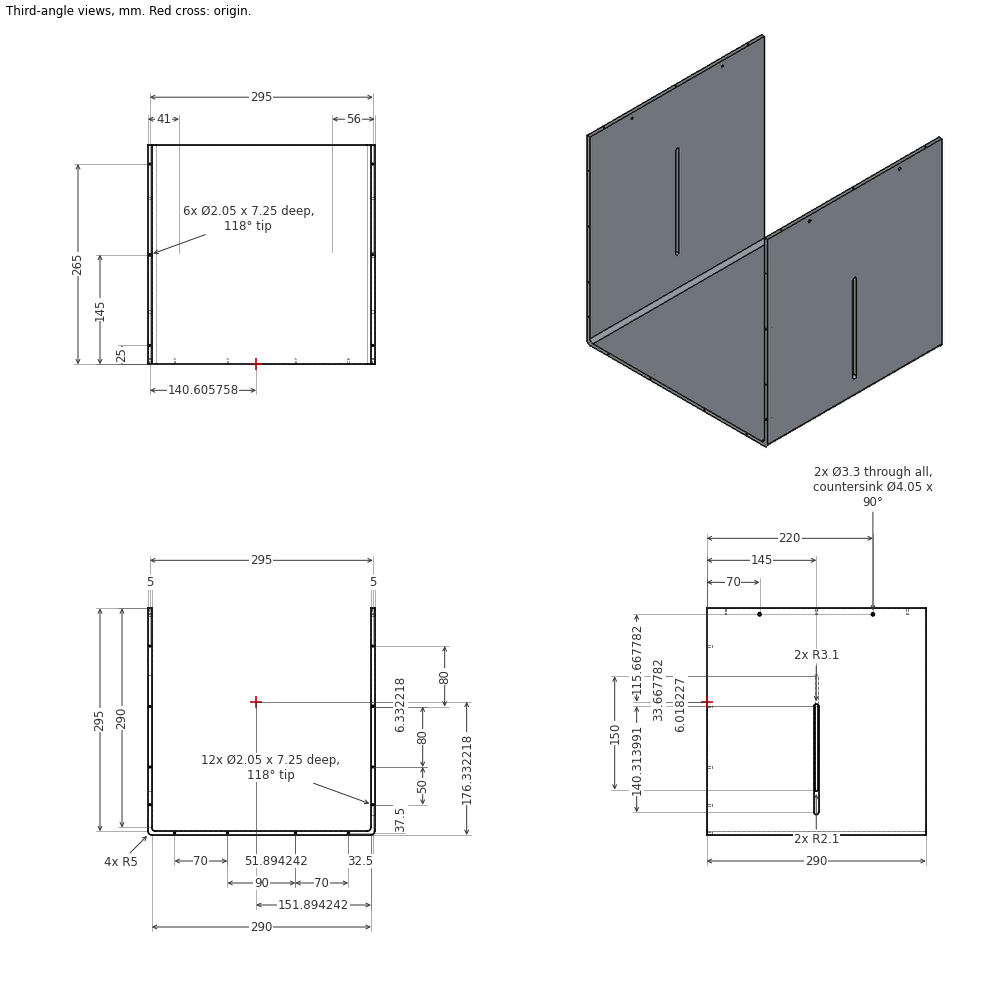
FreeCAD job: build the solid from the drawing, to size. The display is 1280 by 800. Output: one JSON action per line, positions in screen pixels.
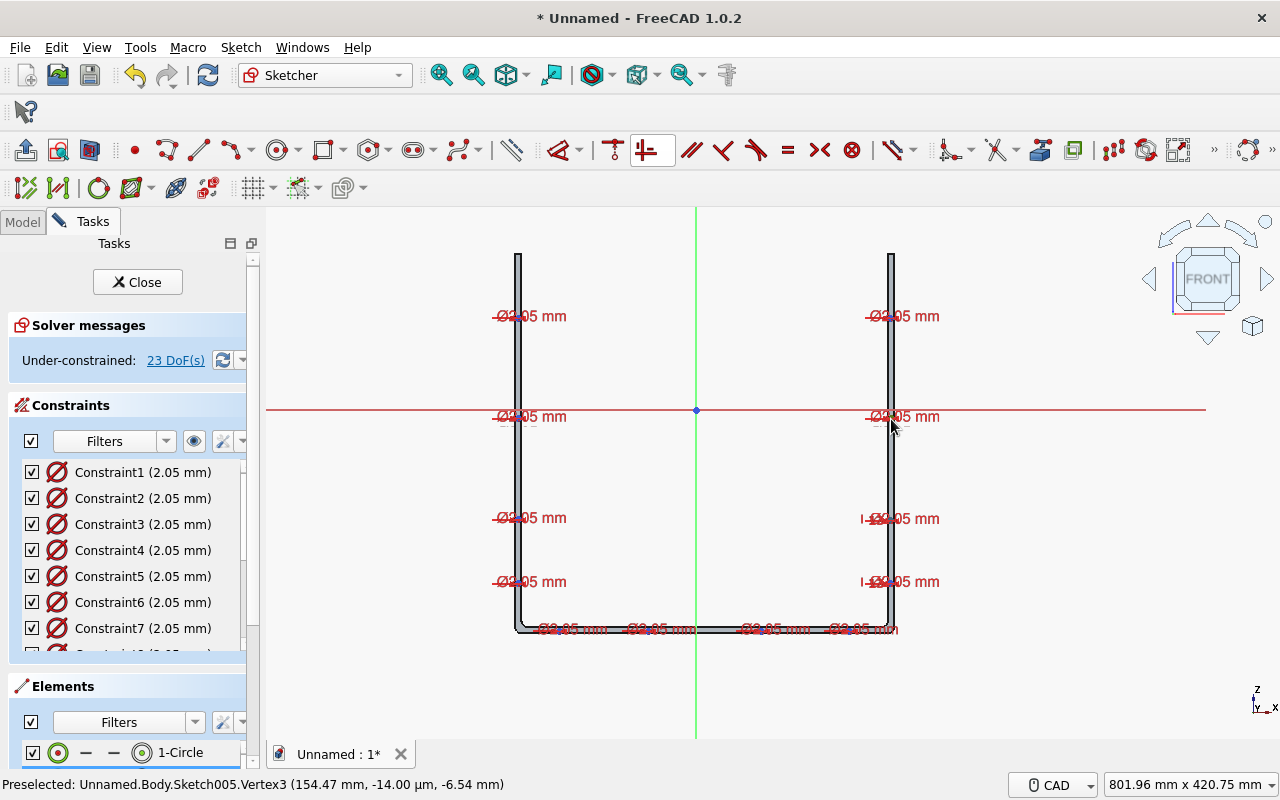
{"action": "key", "text": "v"}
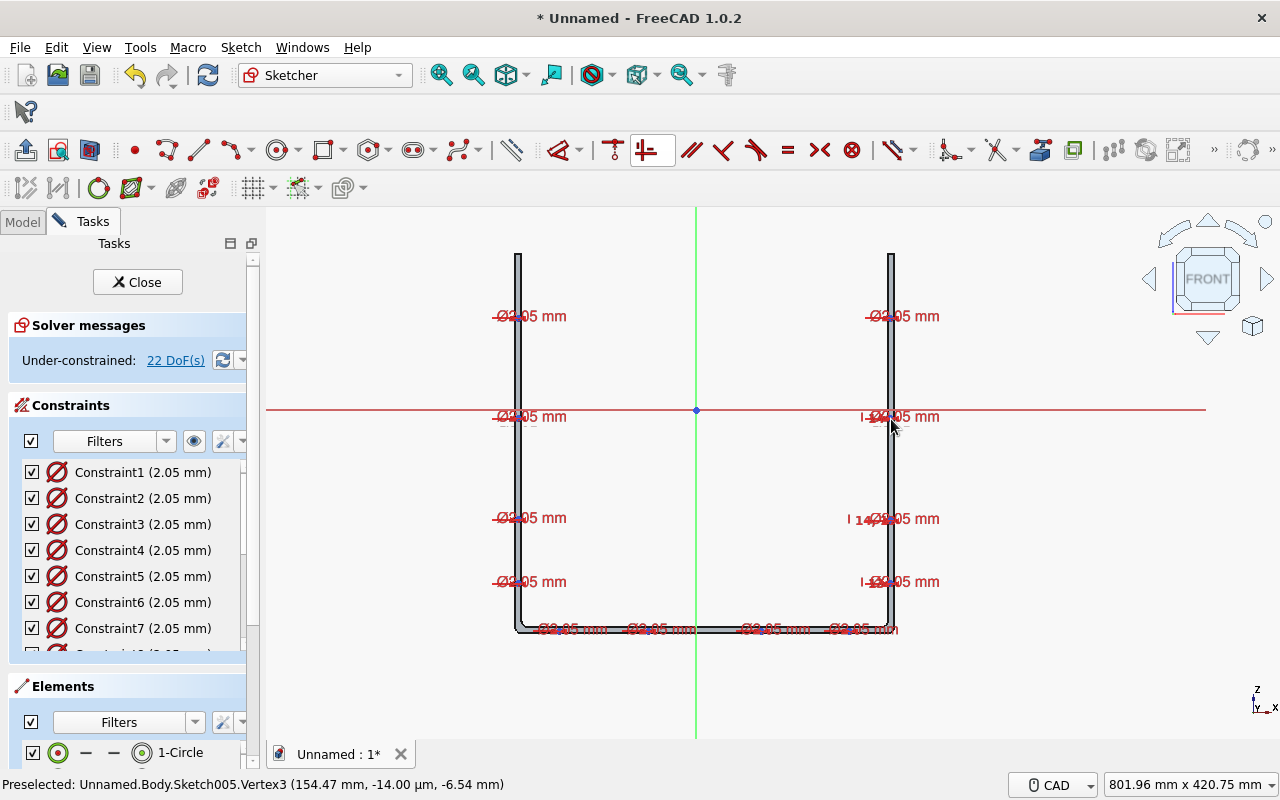
{"action": "left_click", "coordinate": [891, 419]}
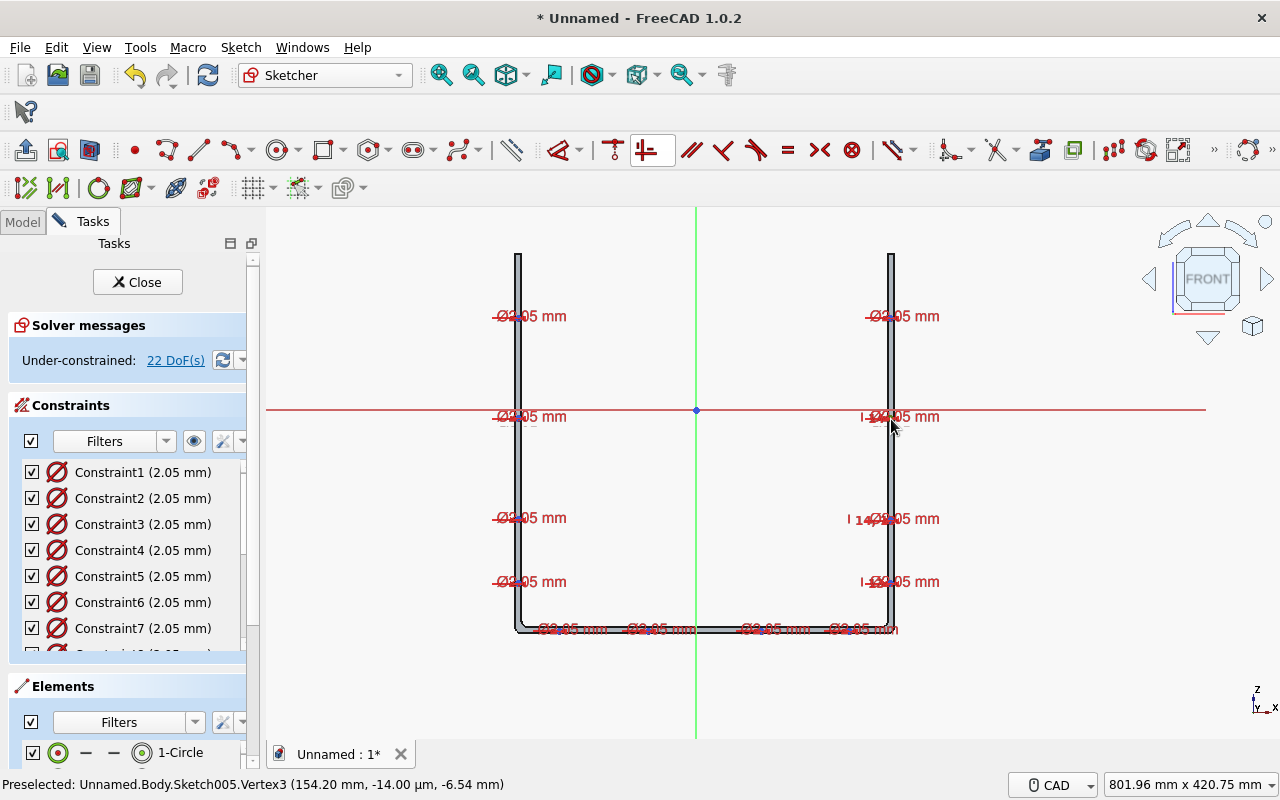
{"action": "left_click", "coordinate": [891, 318]}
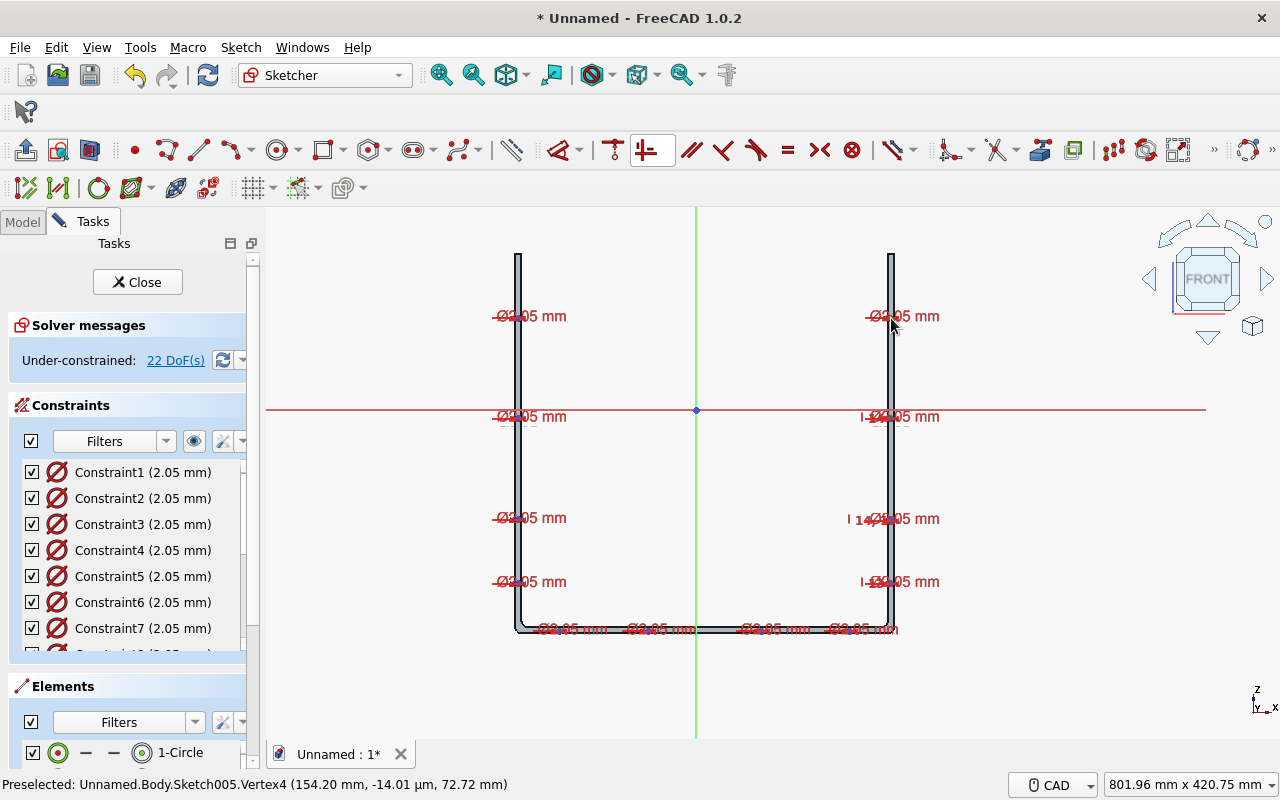
{"action": "left_click", "coordinate": [670, 150]}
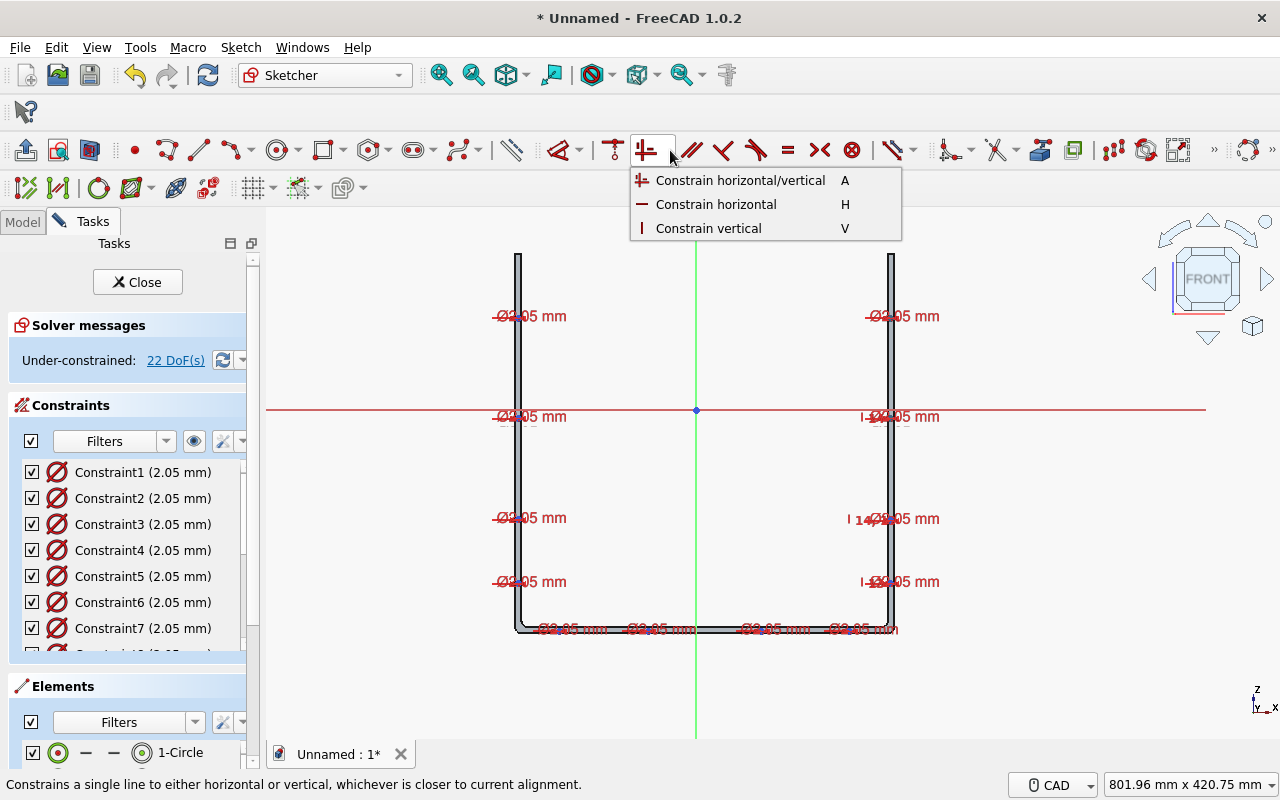
{"action": "left_click", "coordinate": [766, 228]}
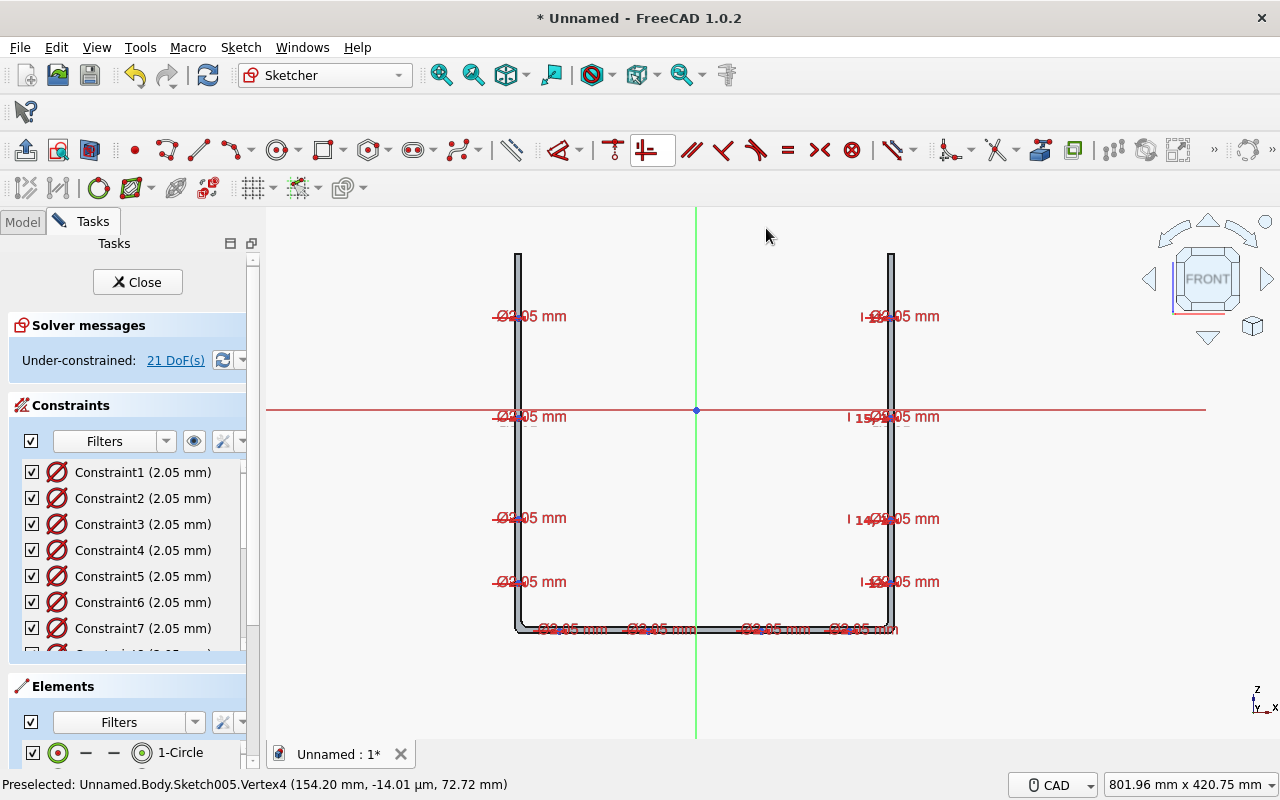
{"action": "left_click", "coordinate": [850, 631]}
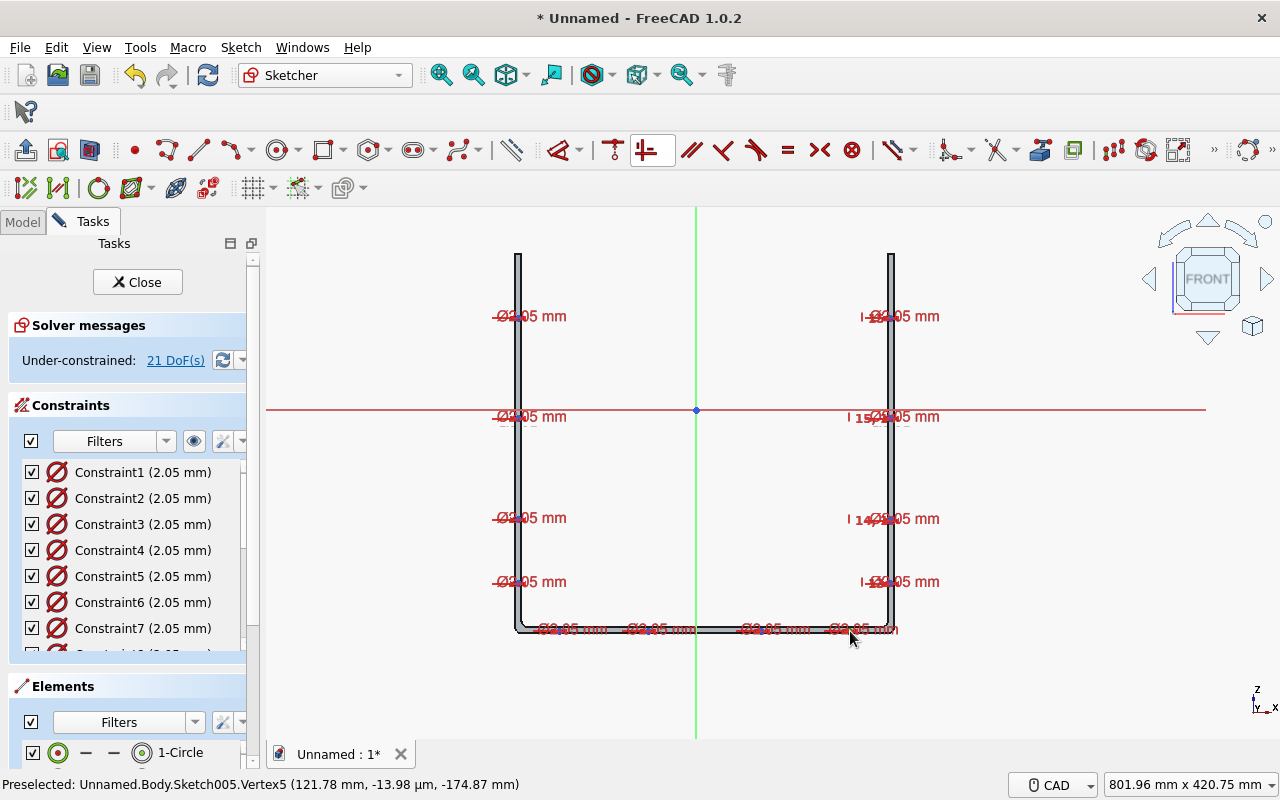
{"action": "left_click", "coordinate": [762, 631]}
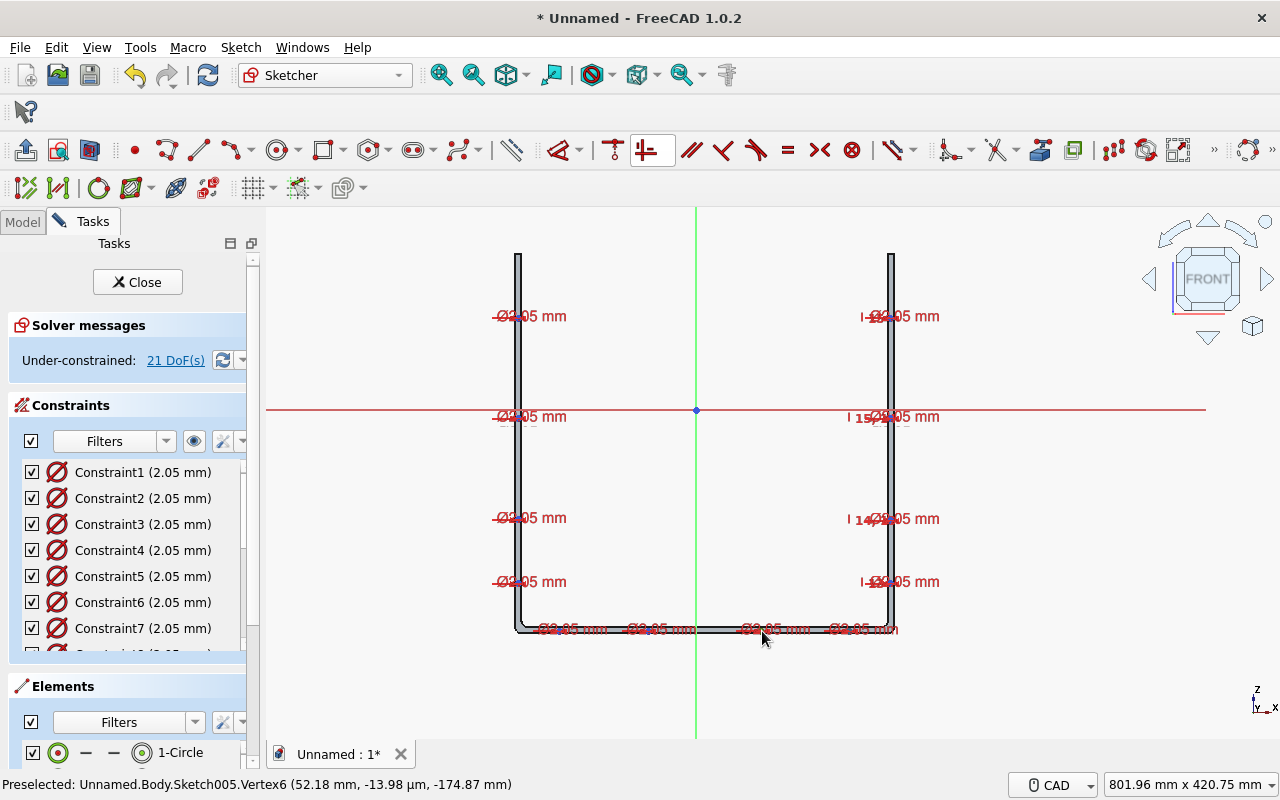
{"action": "left_click", "coordinate": [670, 150]}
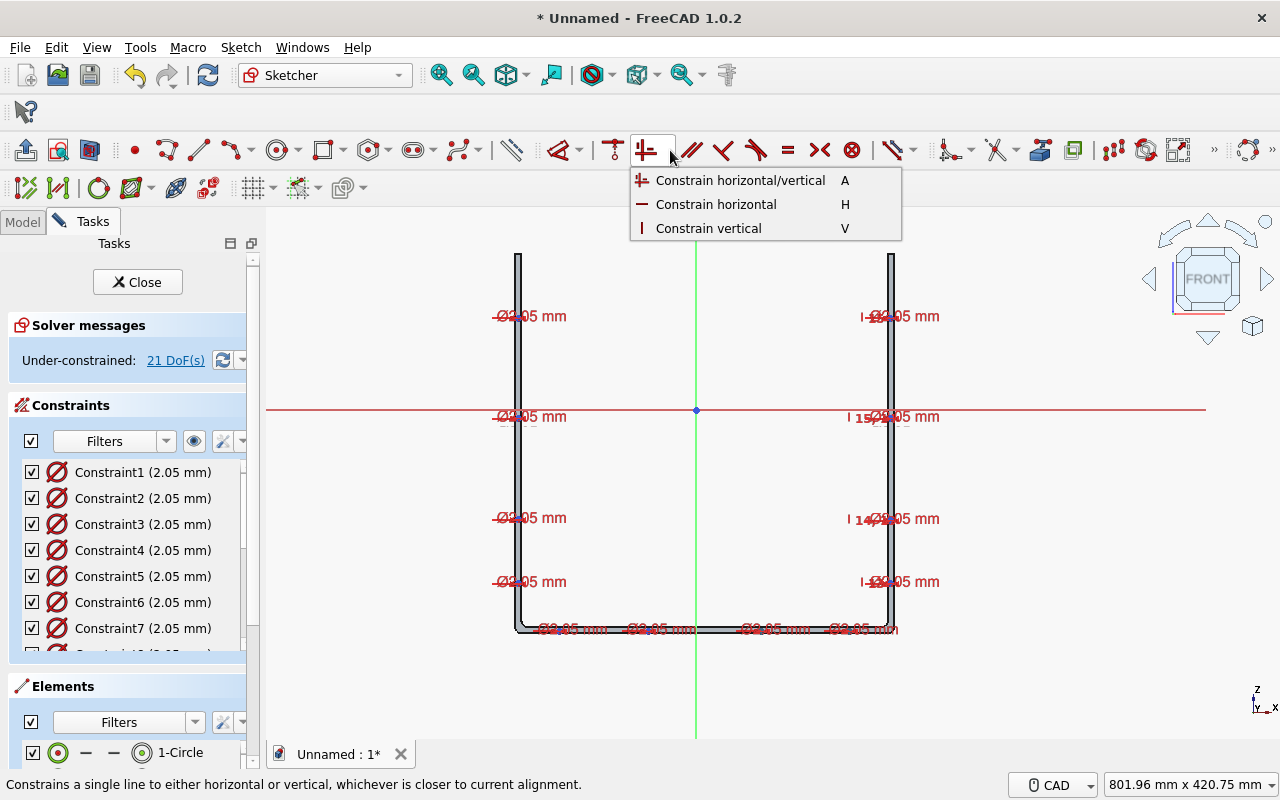
{"action": "left_click", "coordinate": [766, 204]}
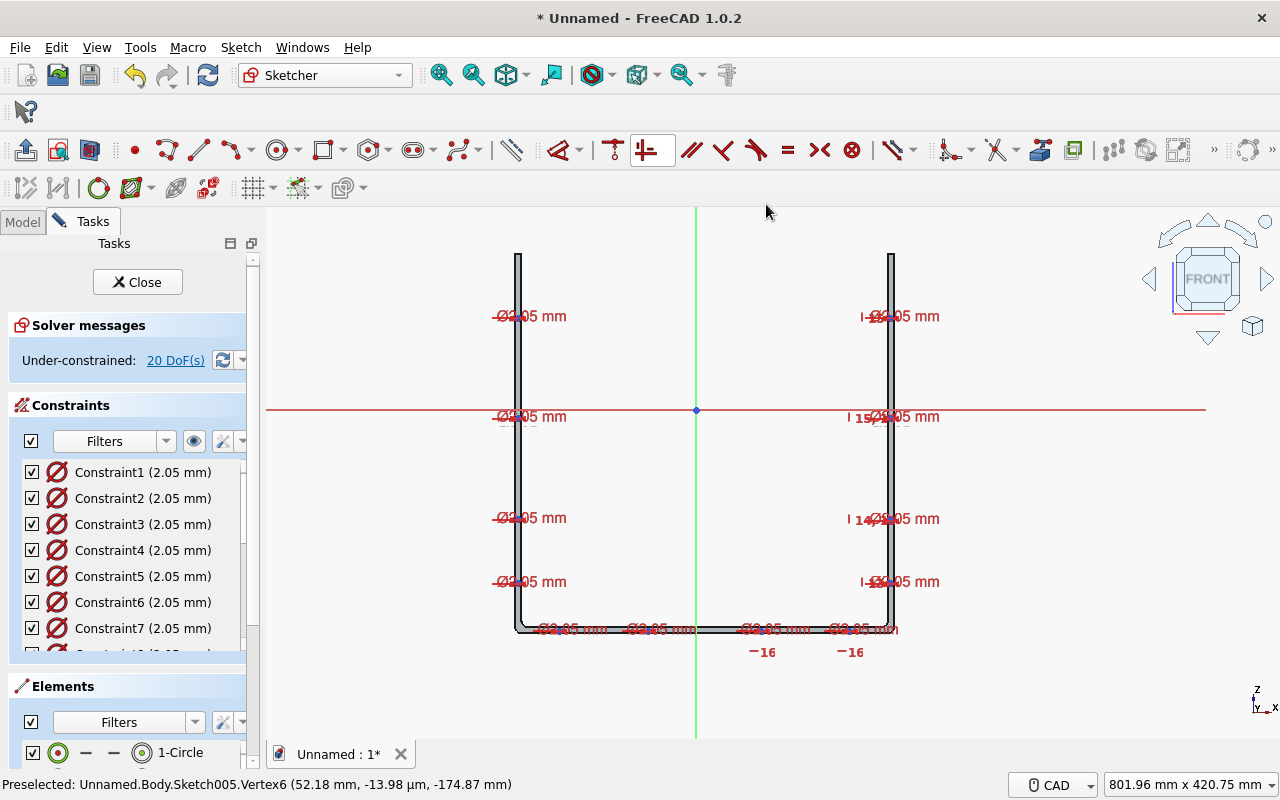
{"action": "left_click", "coordinate": [762, 631]}